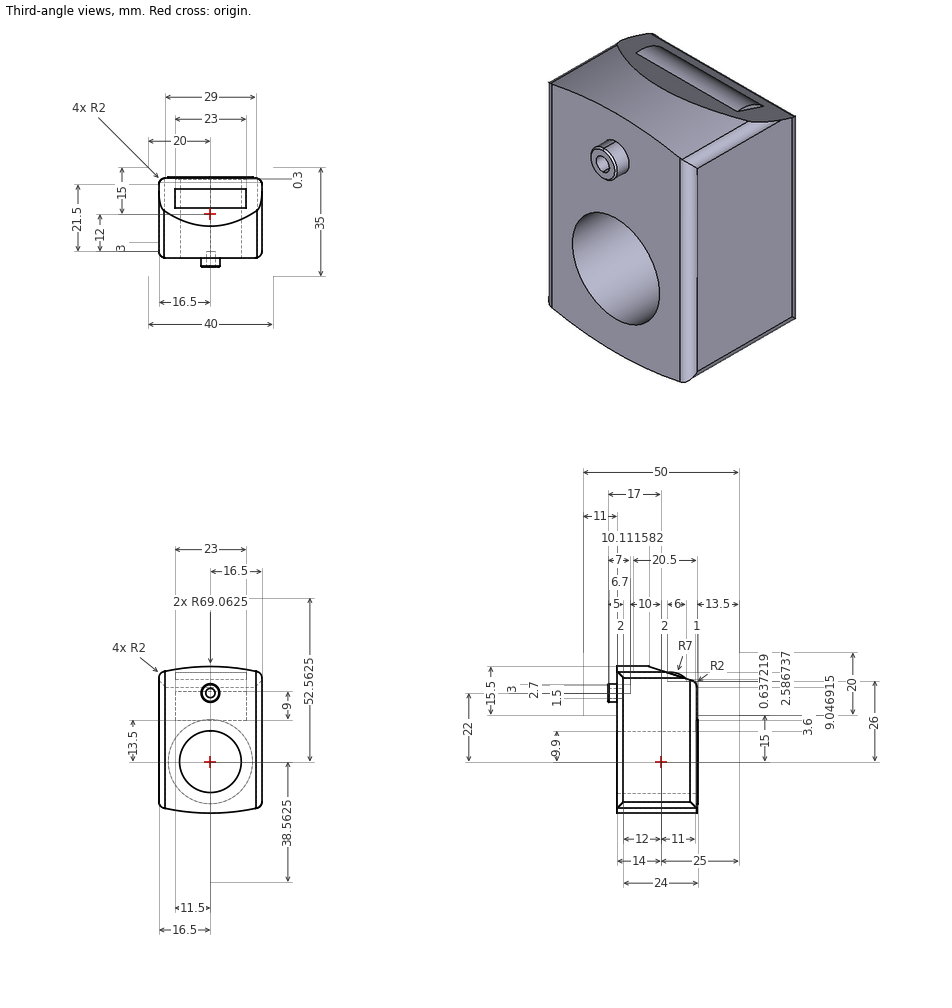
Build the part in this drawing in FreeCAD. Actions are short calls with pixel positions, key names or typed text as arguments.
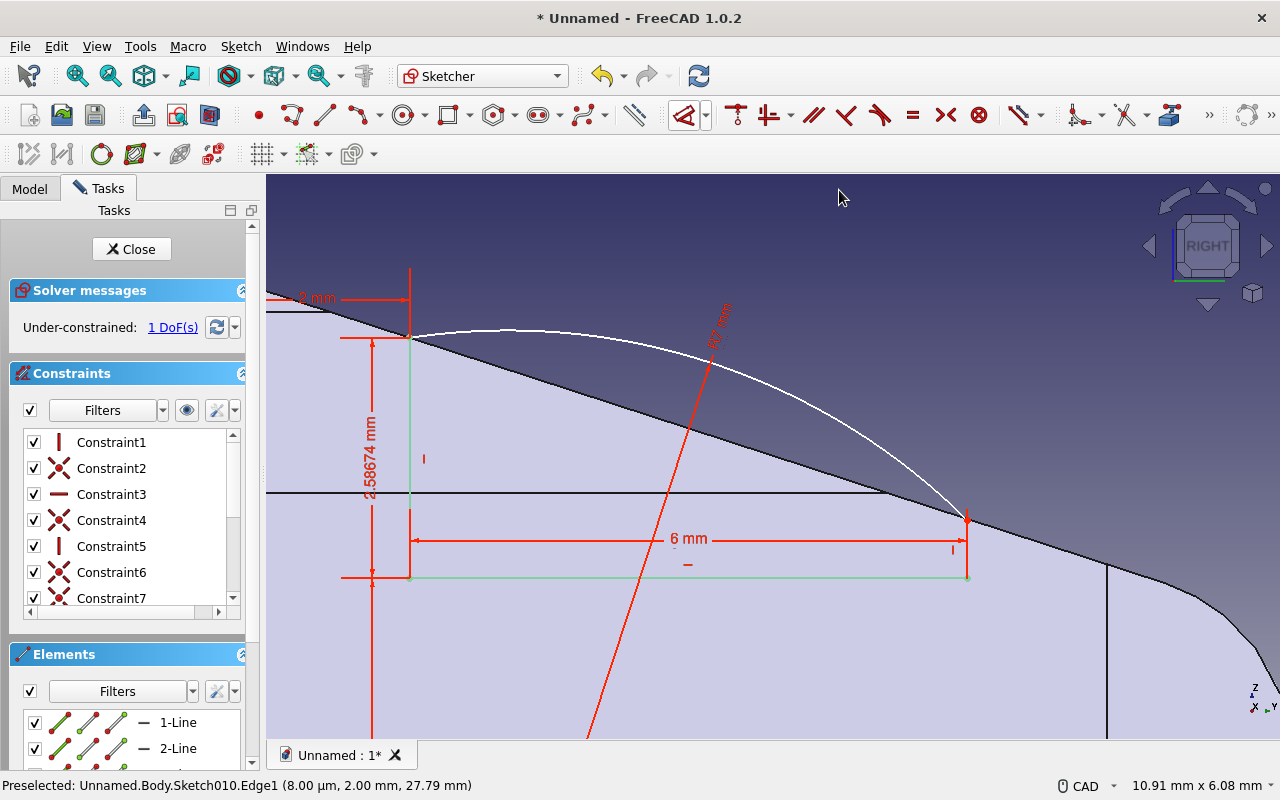
click(967, 561)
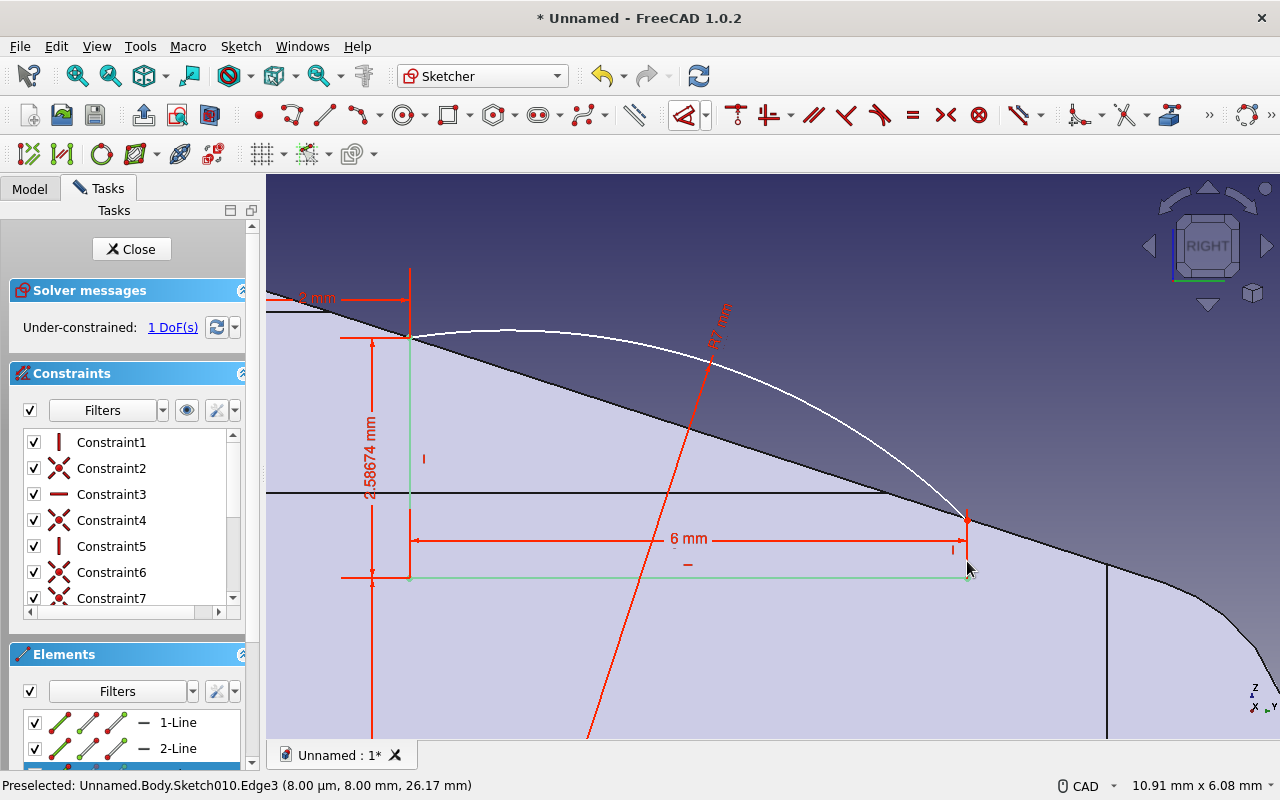
click(706, 116)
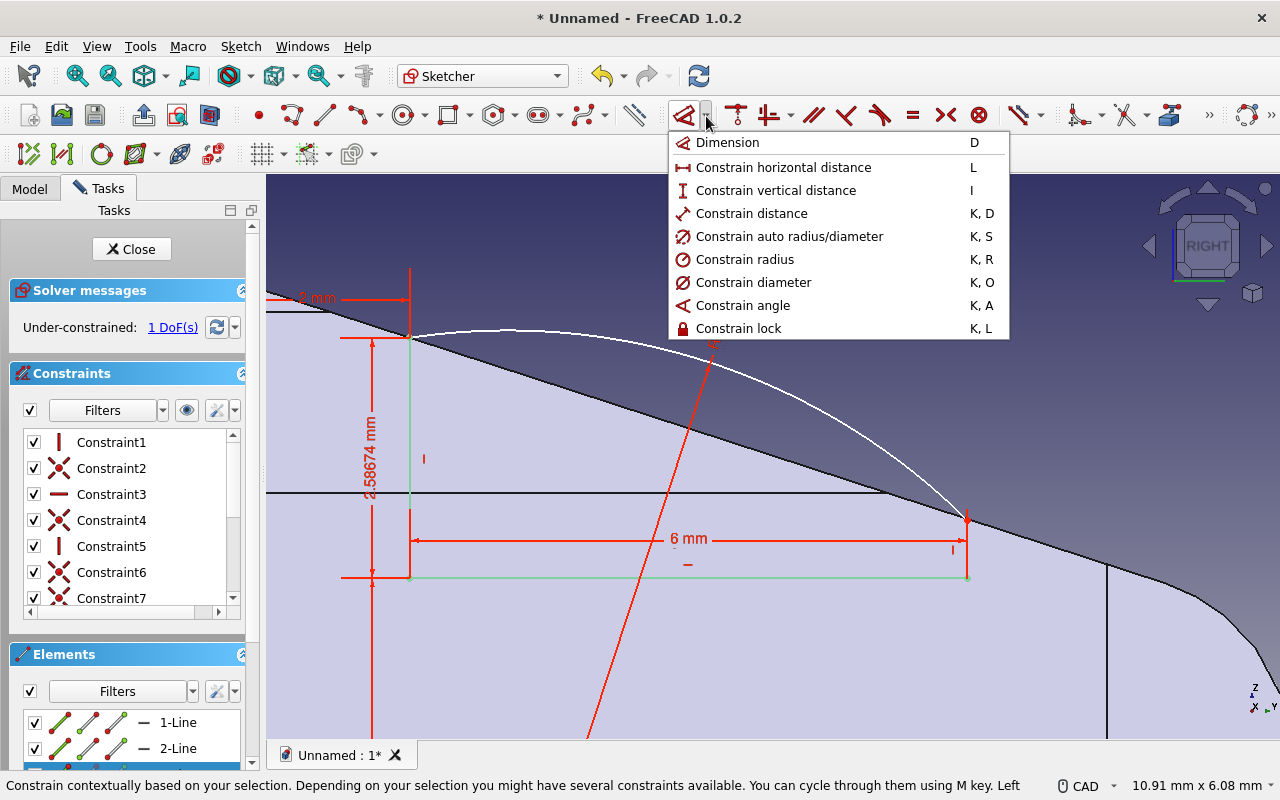
click(839, 190)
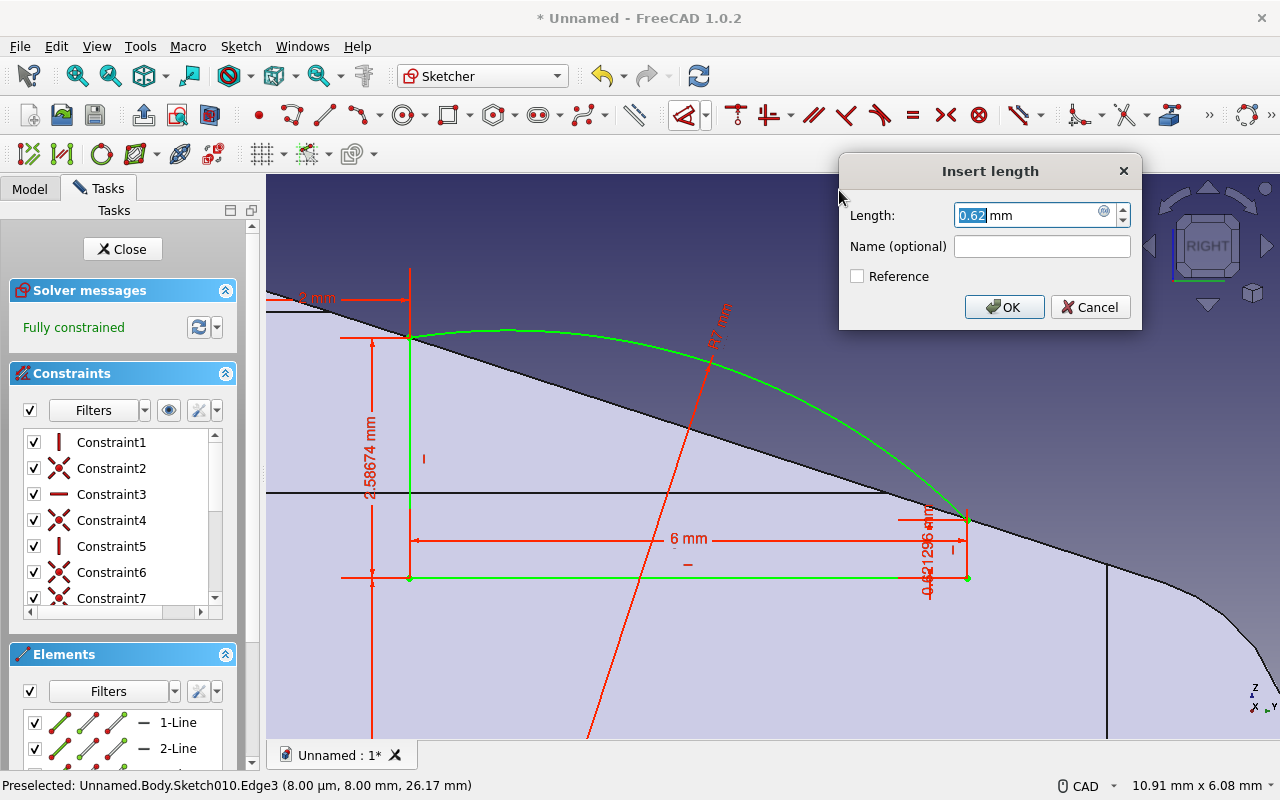
text(0.637219)
key(Return)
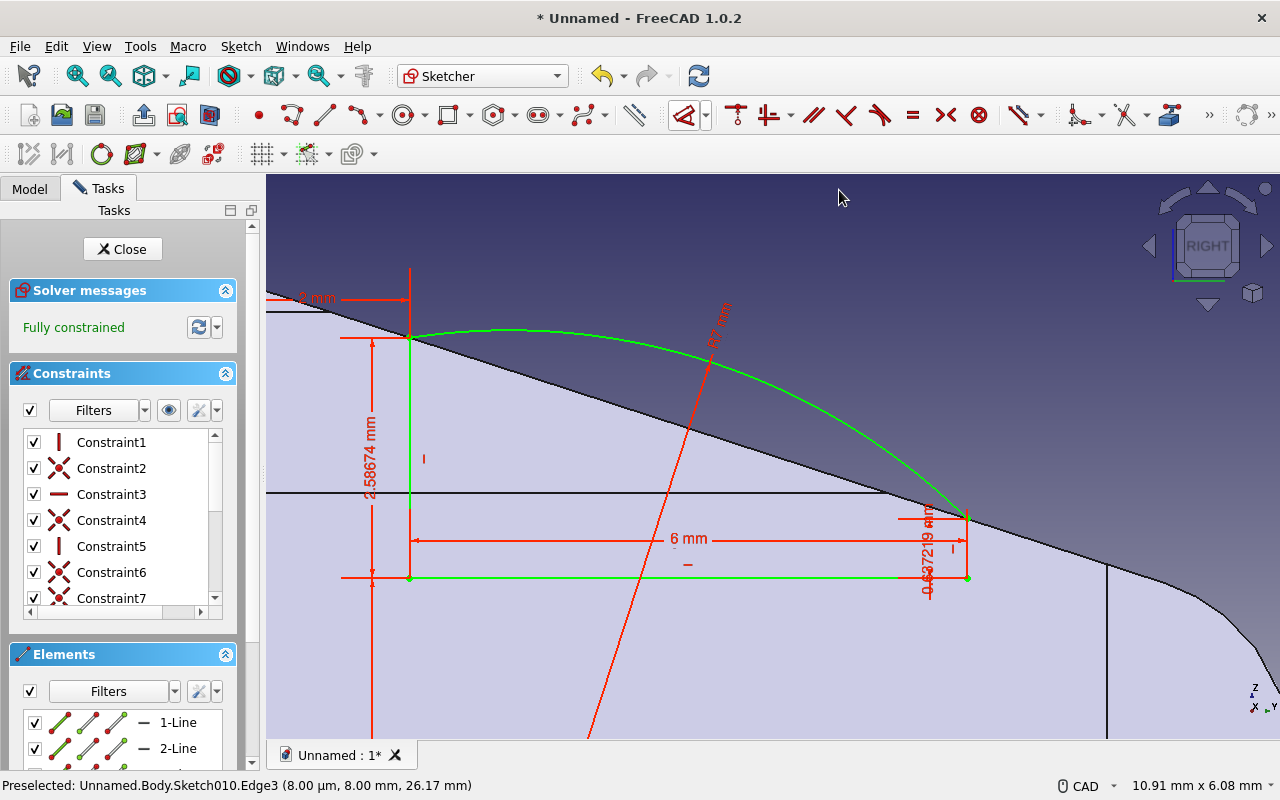
click(123, 249)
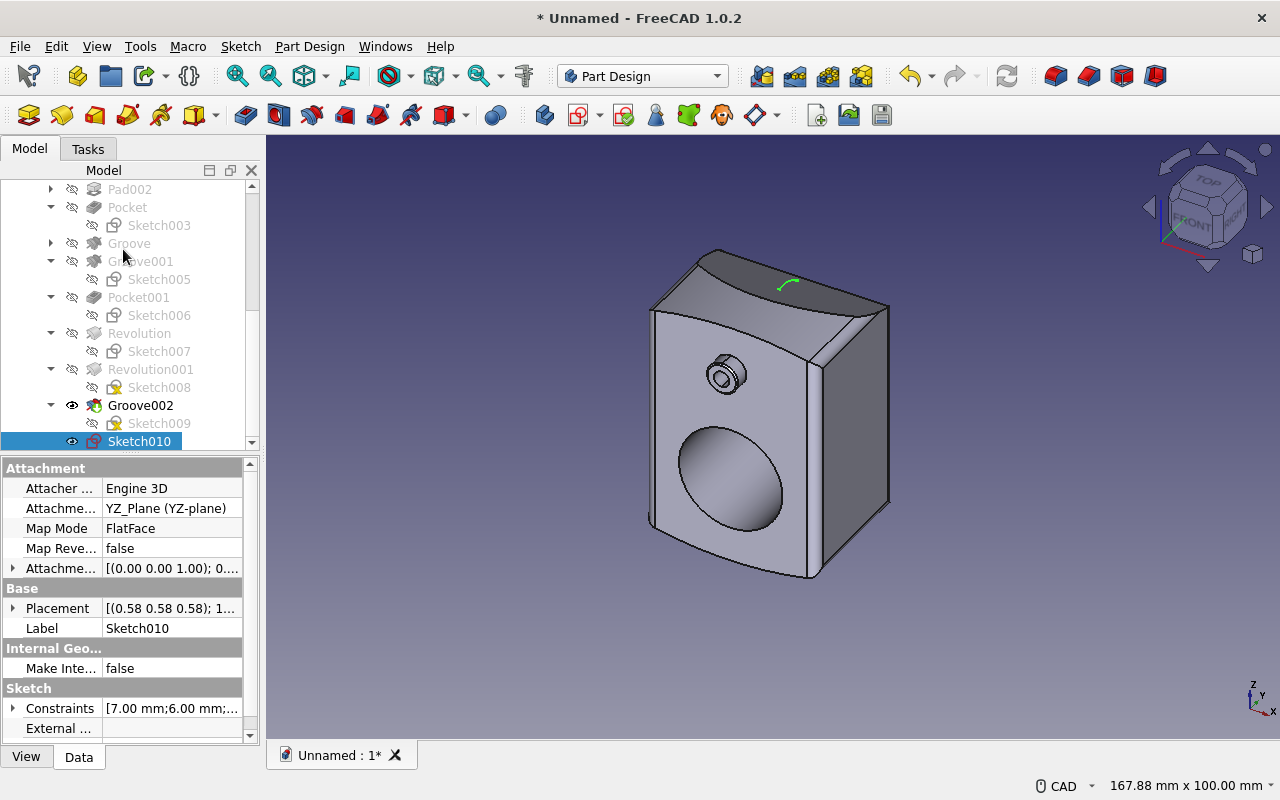
click(29, 116)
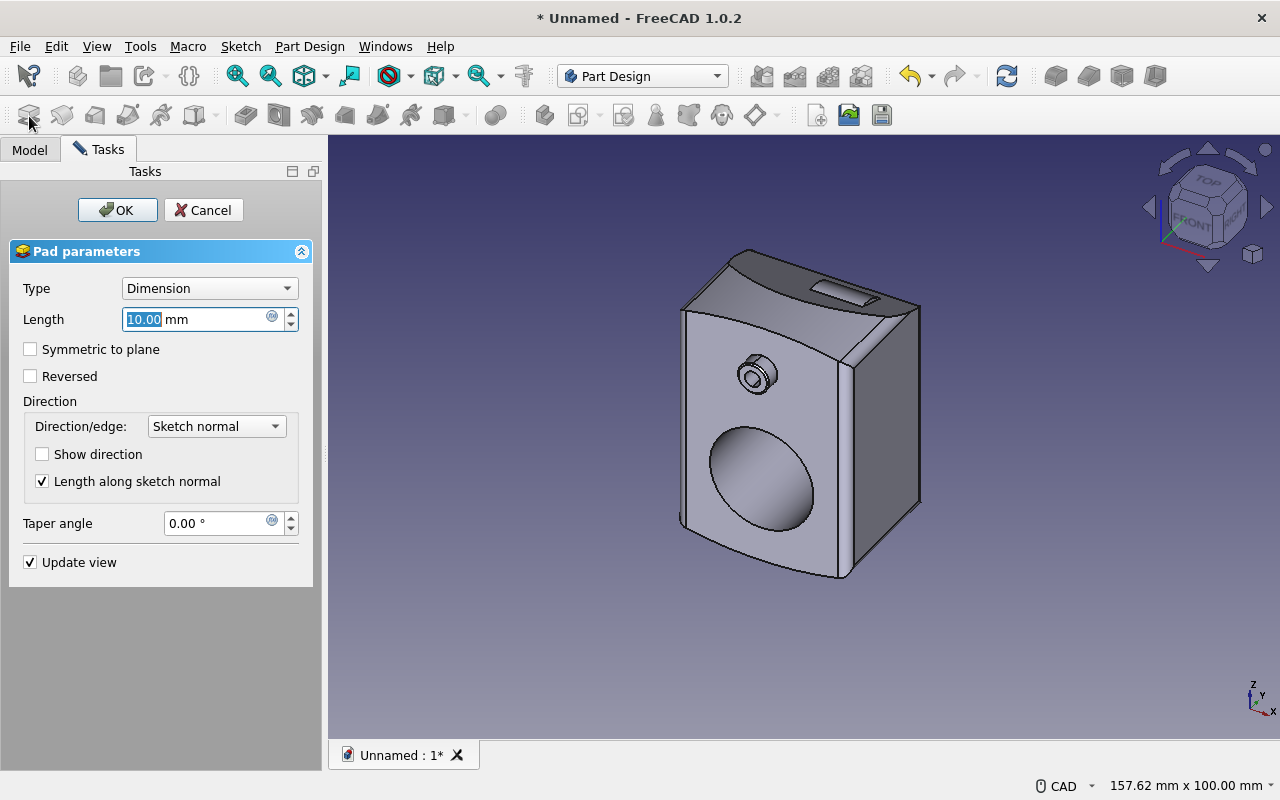
text(23)
key(Tab)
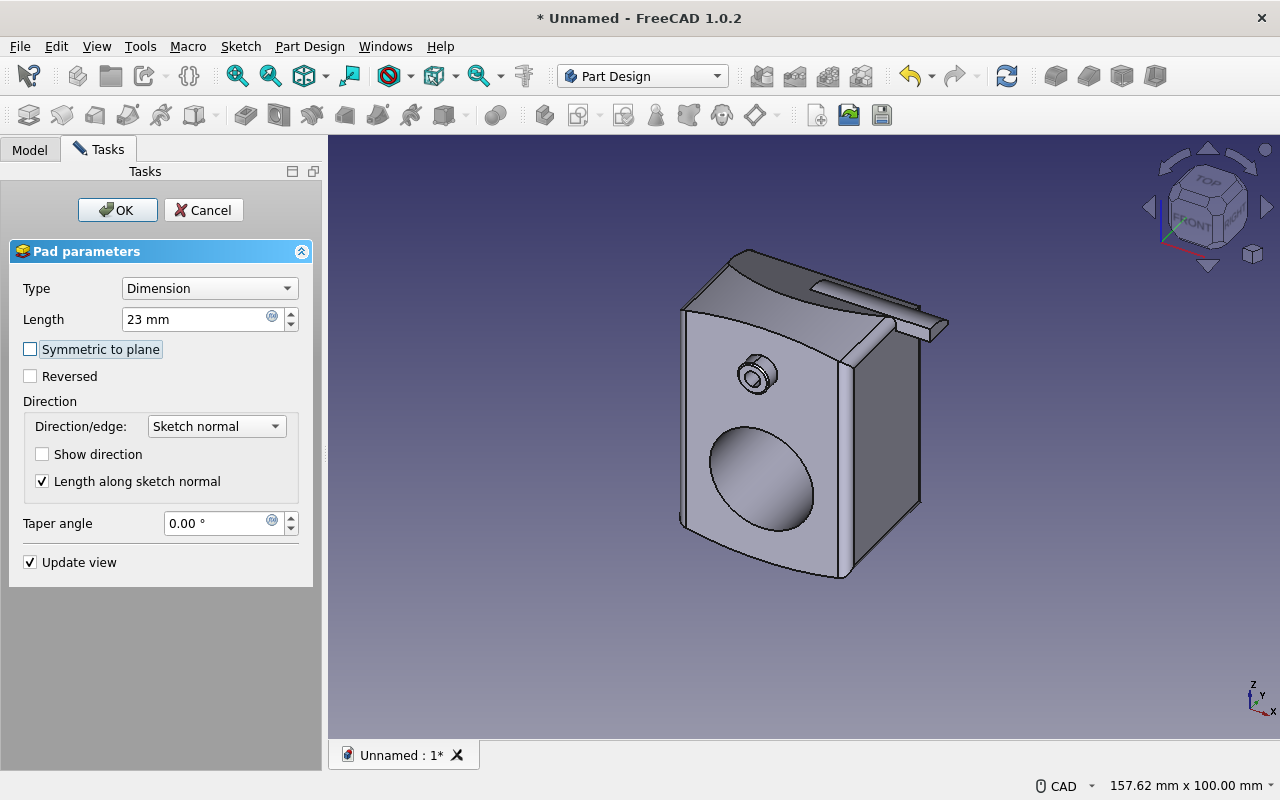
click(31, 349)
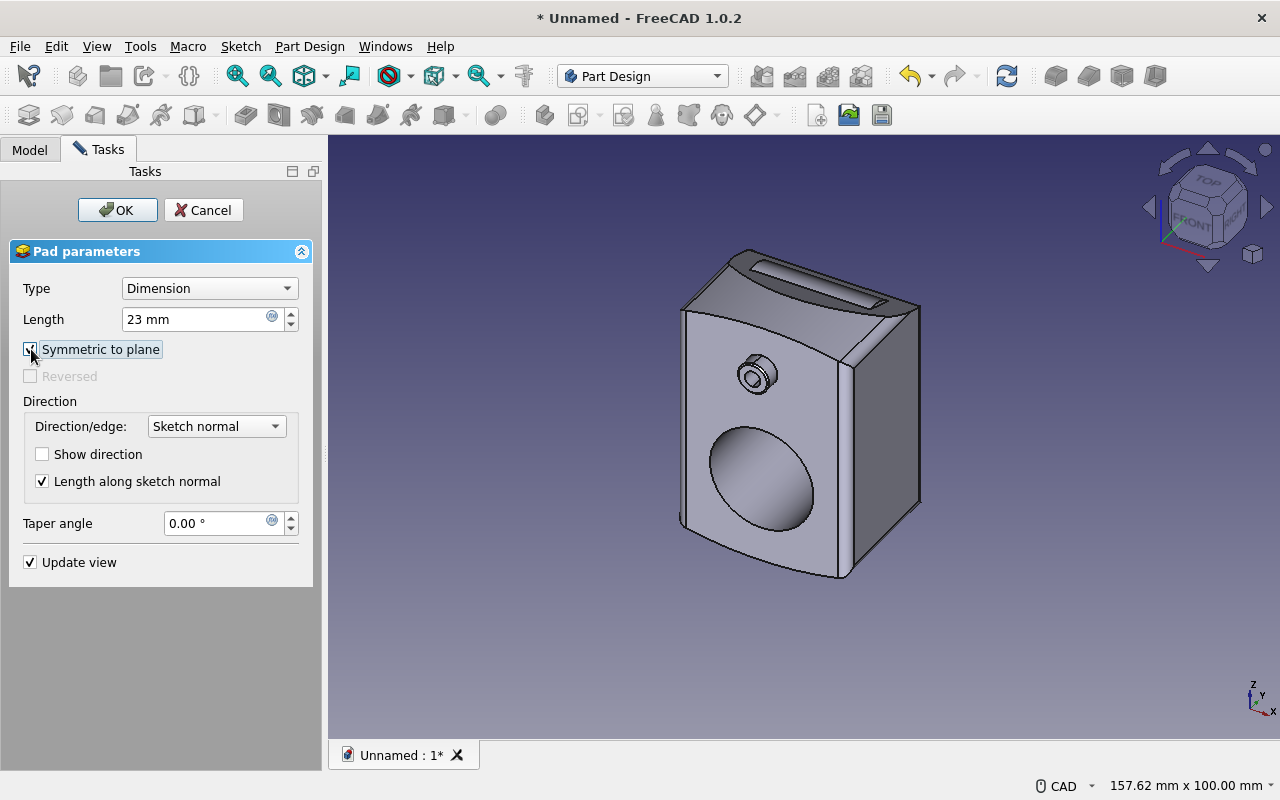
click(118, 210)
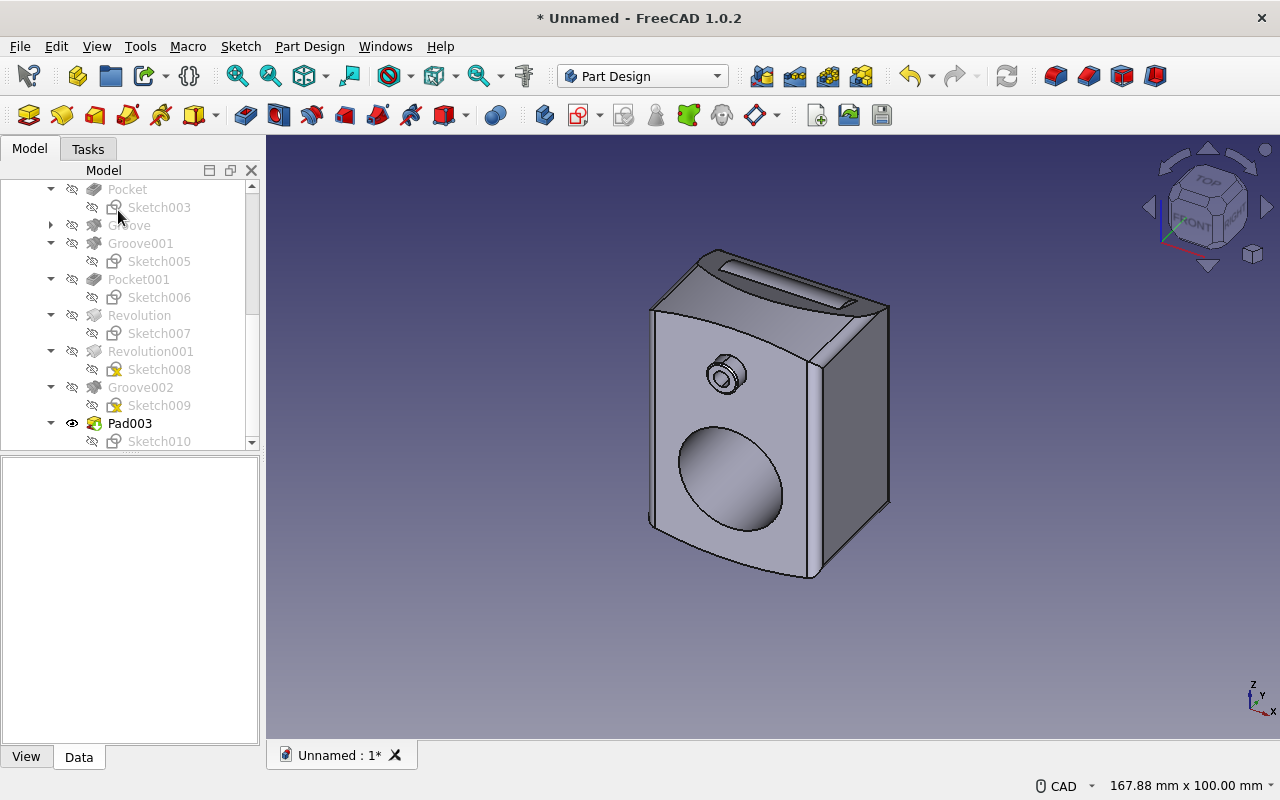
key(4)